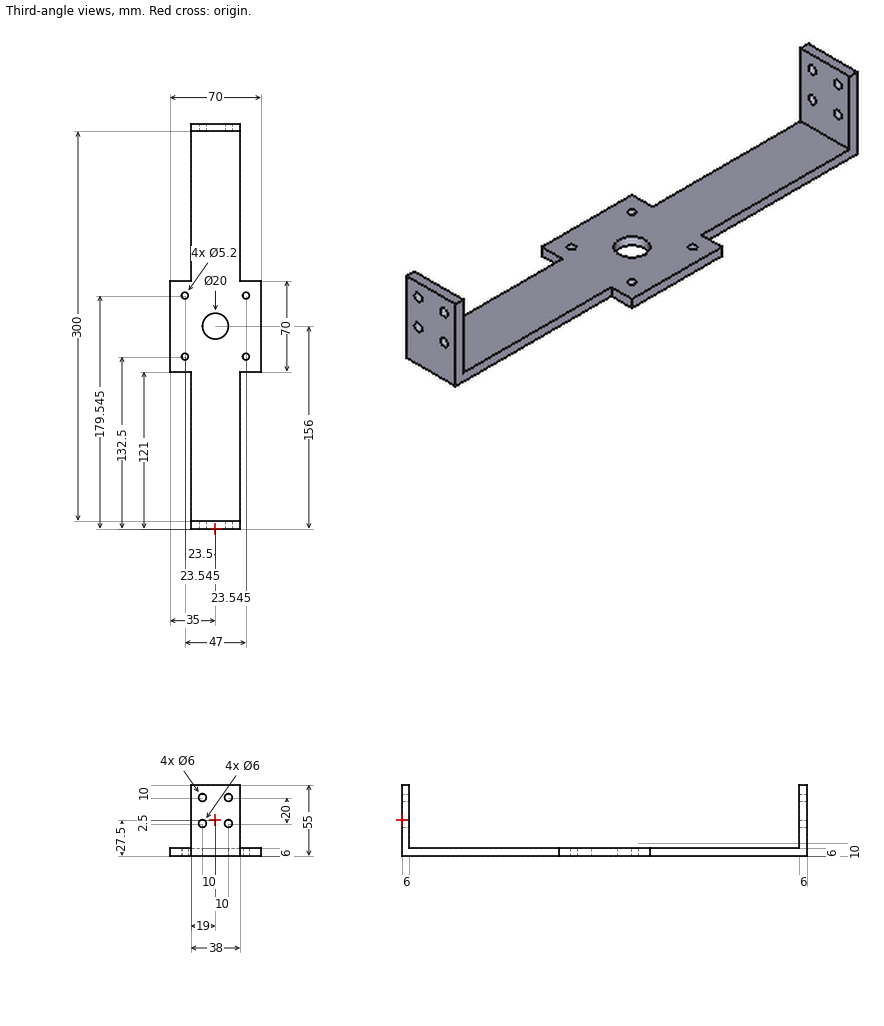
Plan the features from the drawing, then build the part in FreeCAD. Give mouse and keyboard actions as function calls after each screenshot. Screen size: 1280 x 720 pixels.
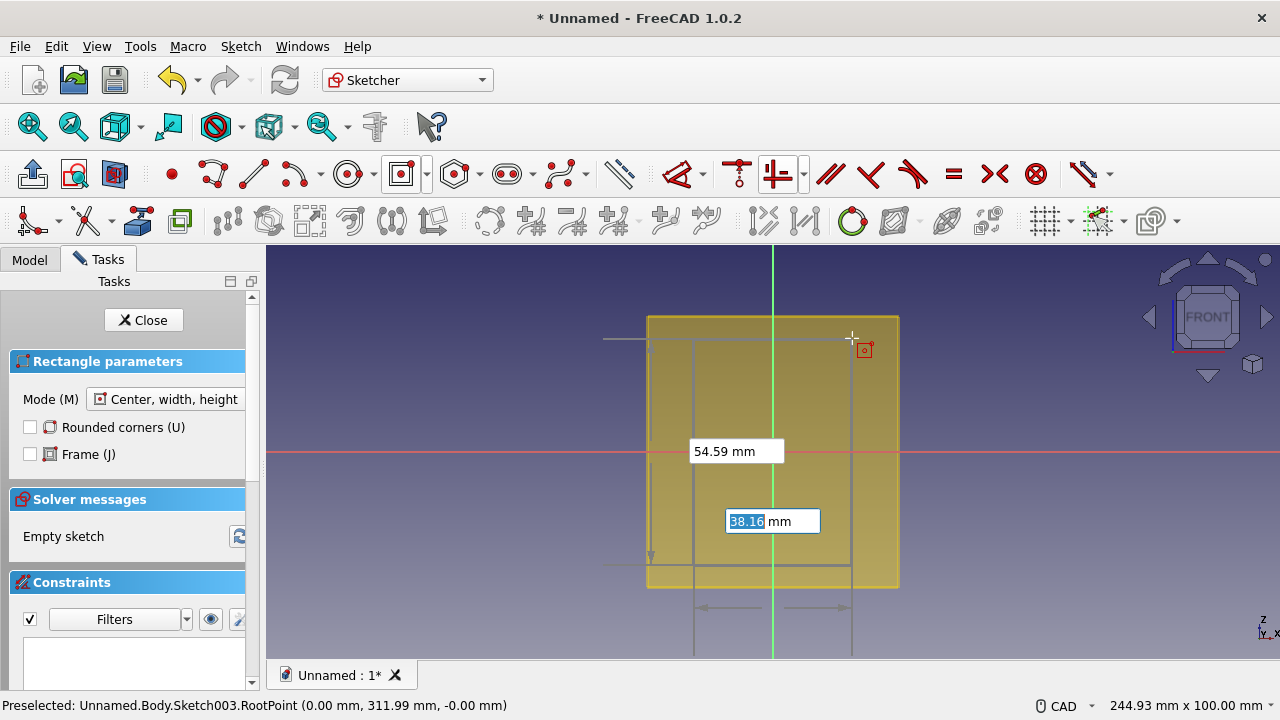
text(38)
key(Tab)
text(55)
key(Return)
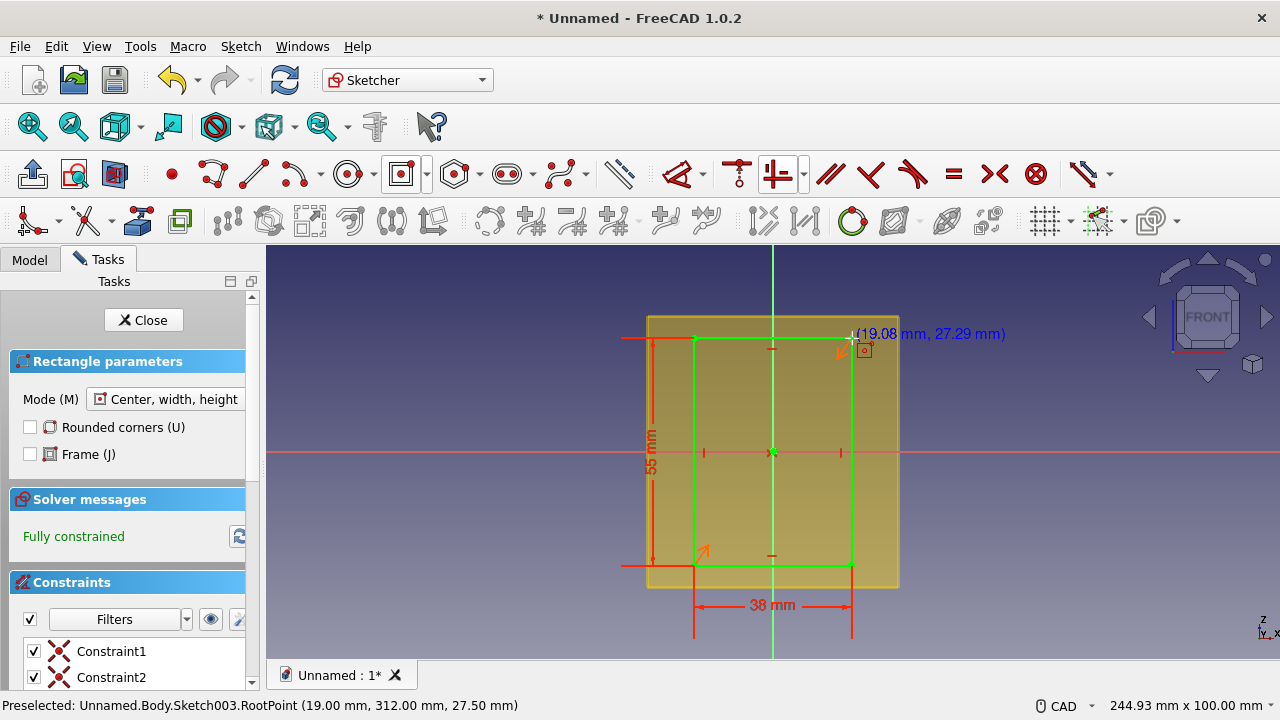
click(348, 174)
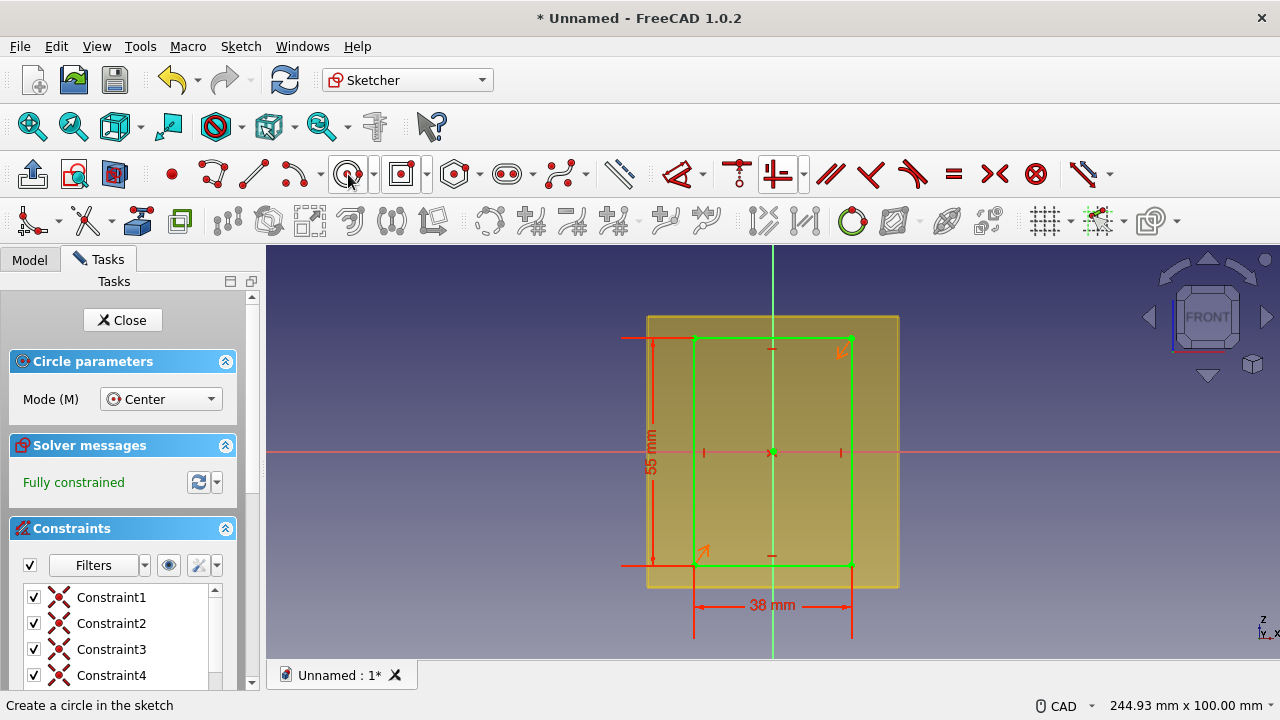
scroll(732, 380, up, 4)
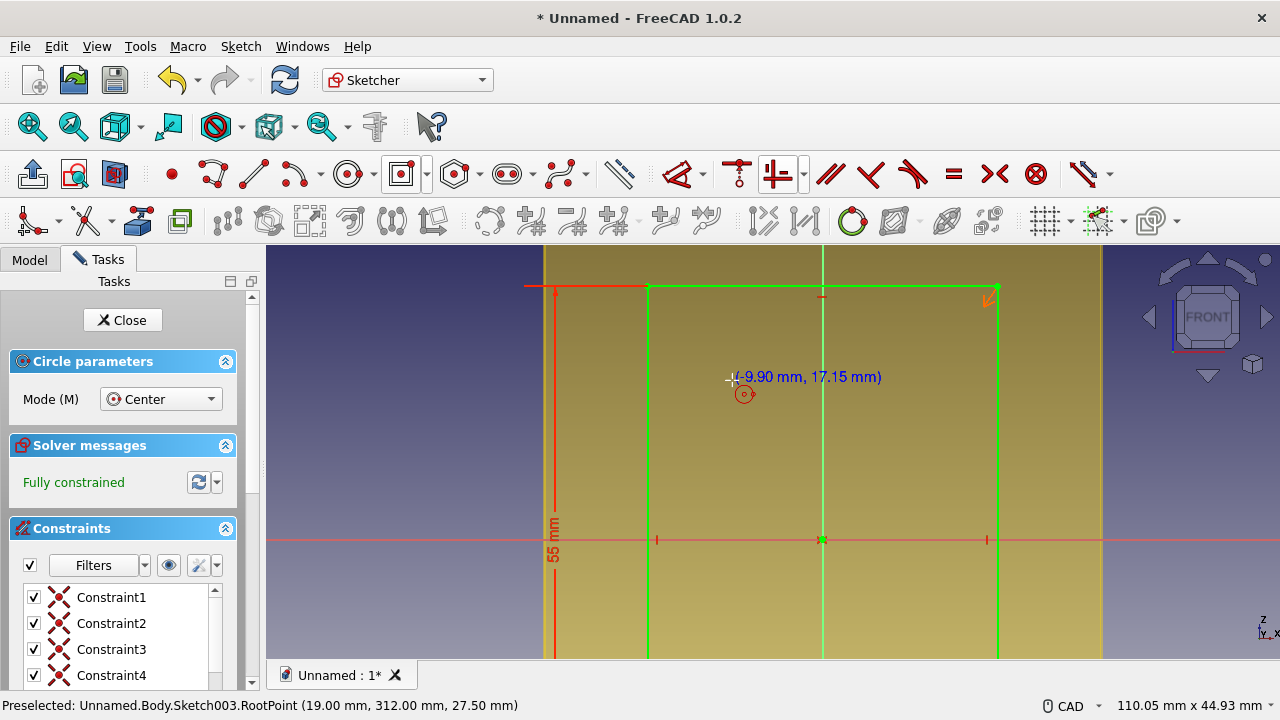
click(731, 379)
move(750, 359)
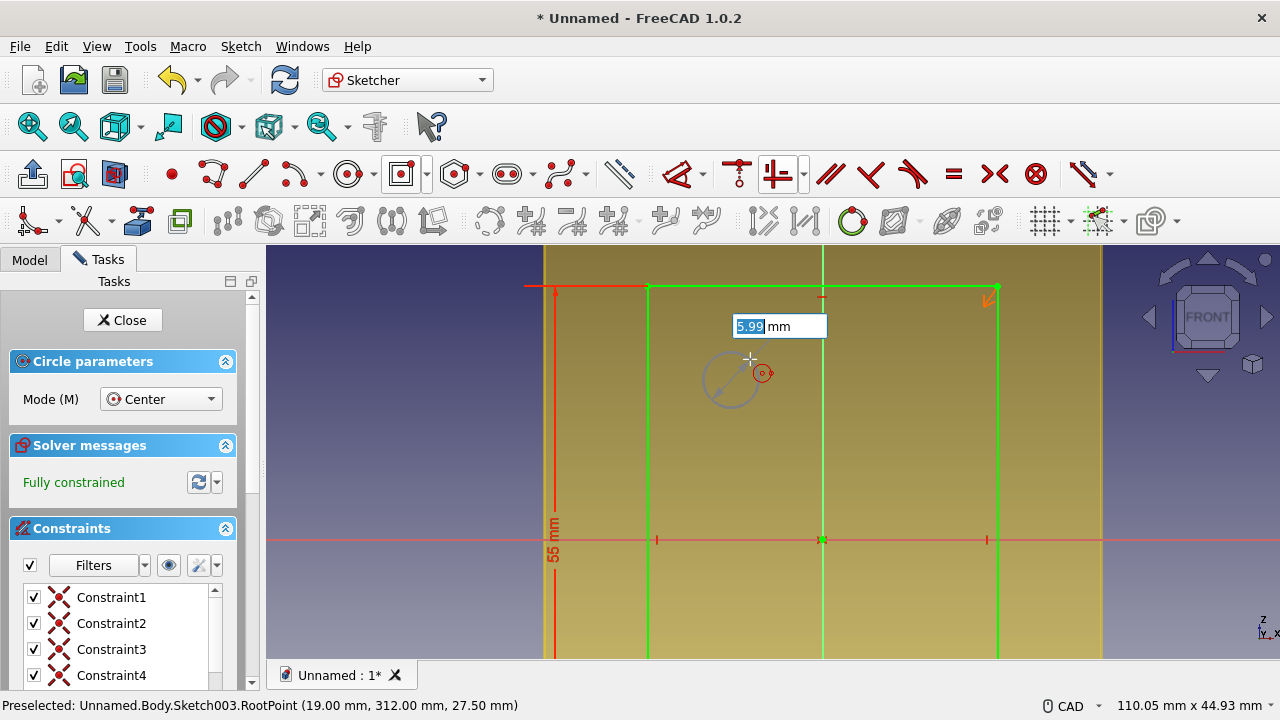
text(6)
key(Return)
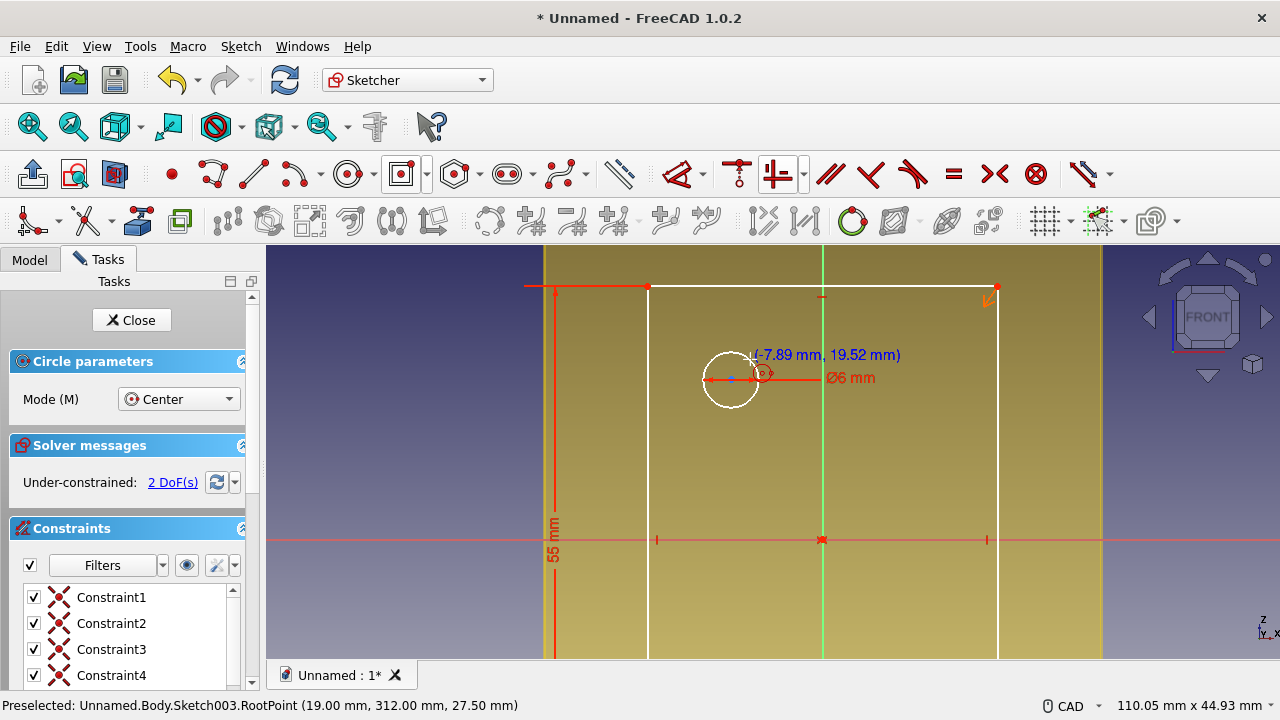
click(915, 379)
move(934, 359)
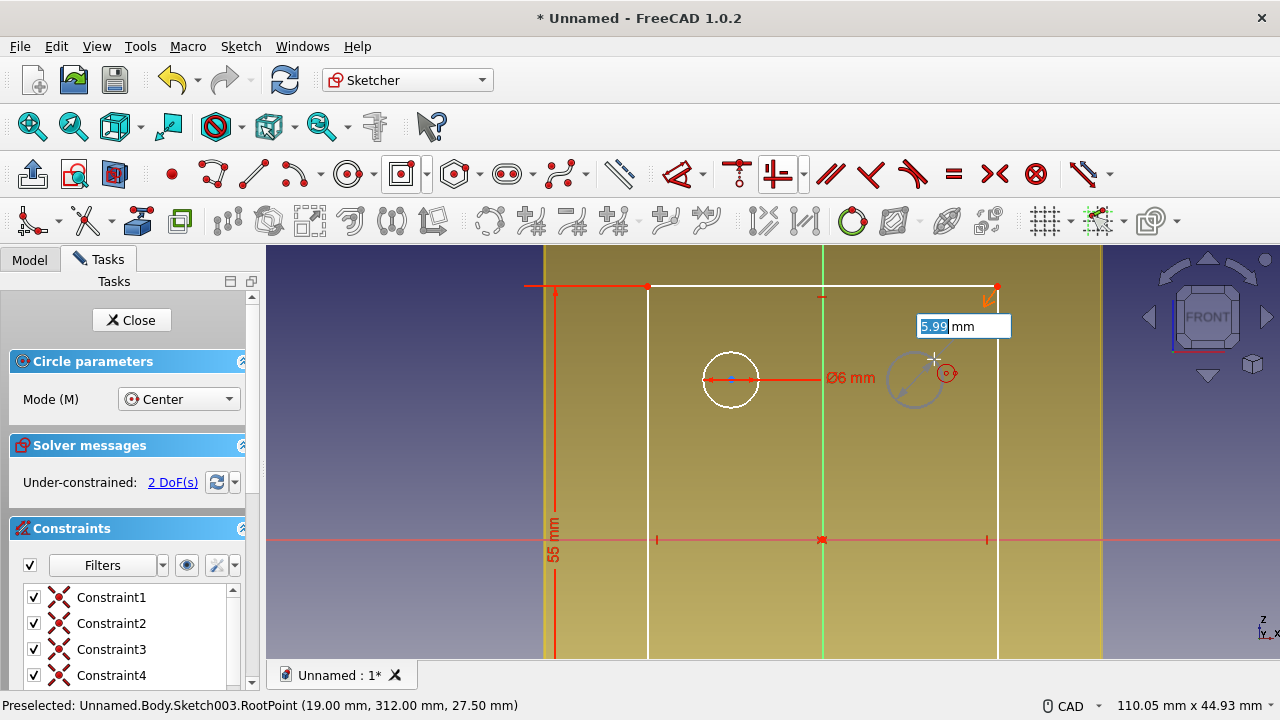
text(6)
key(Return)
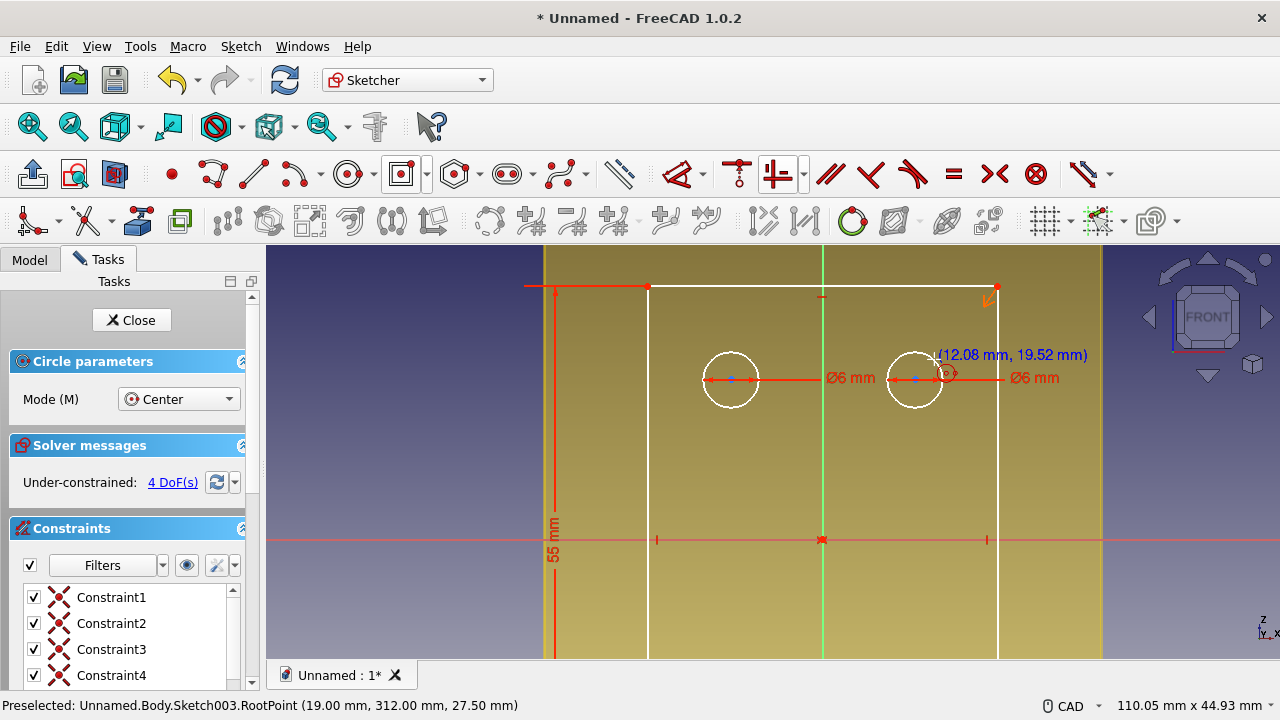
click(731, 563)
move(750, 582)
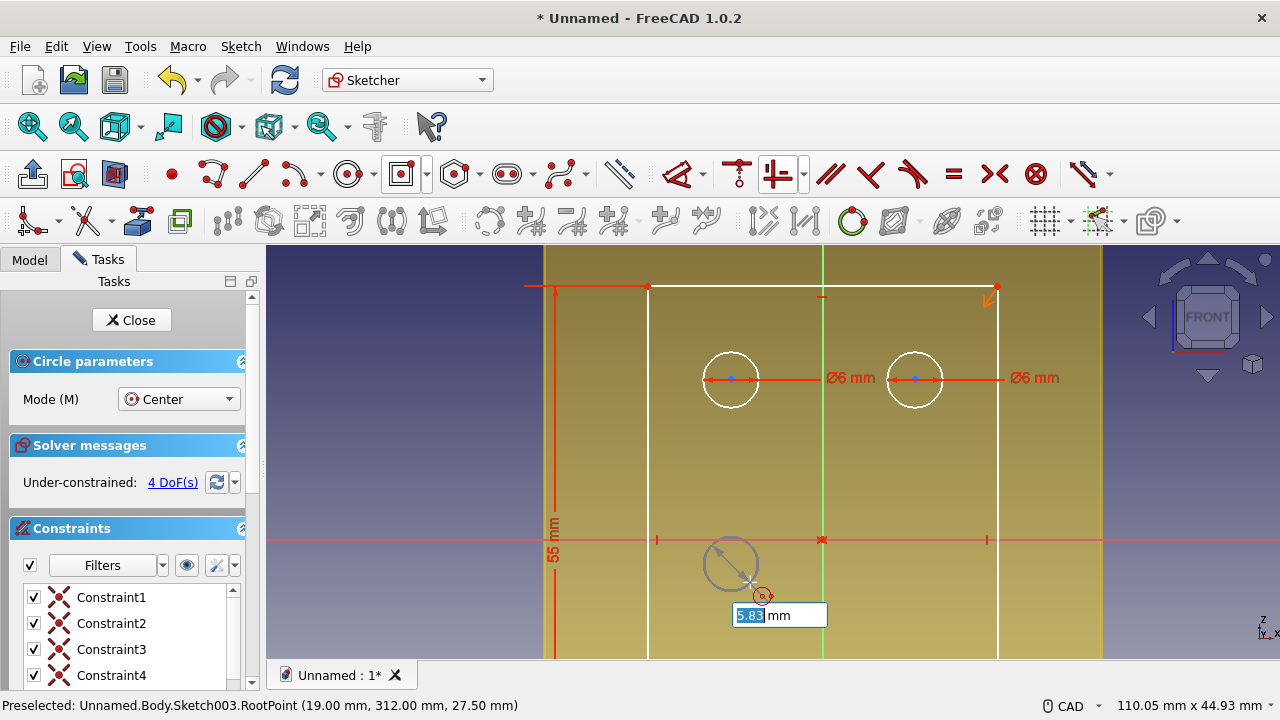
text(6)
key(Return)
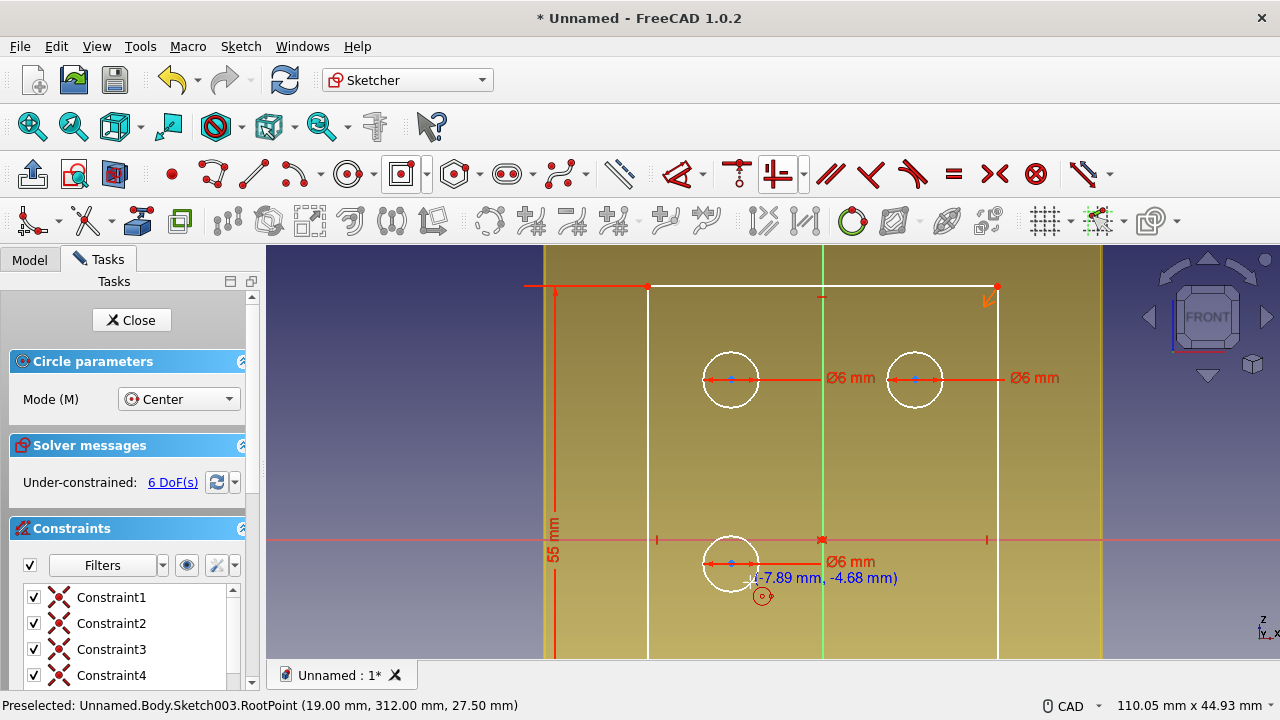
click(915, 563)
move(934, 582)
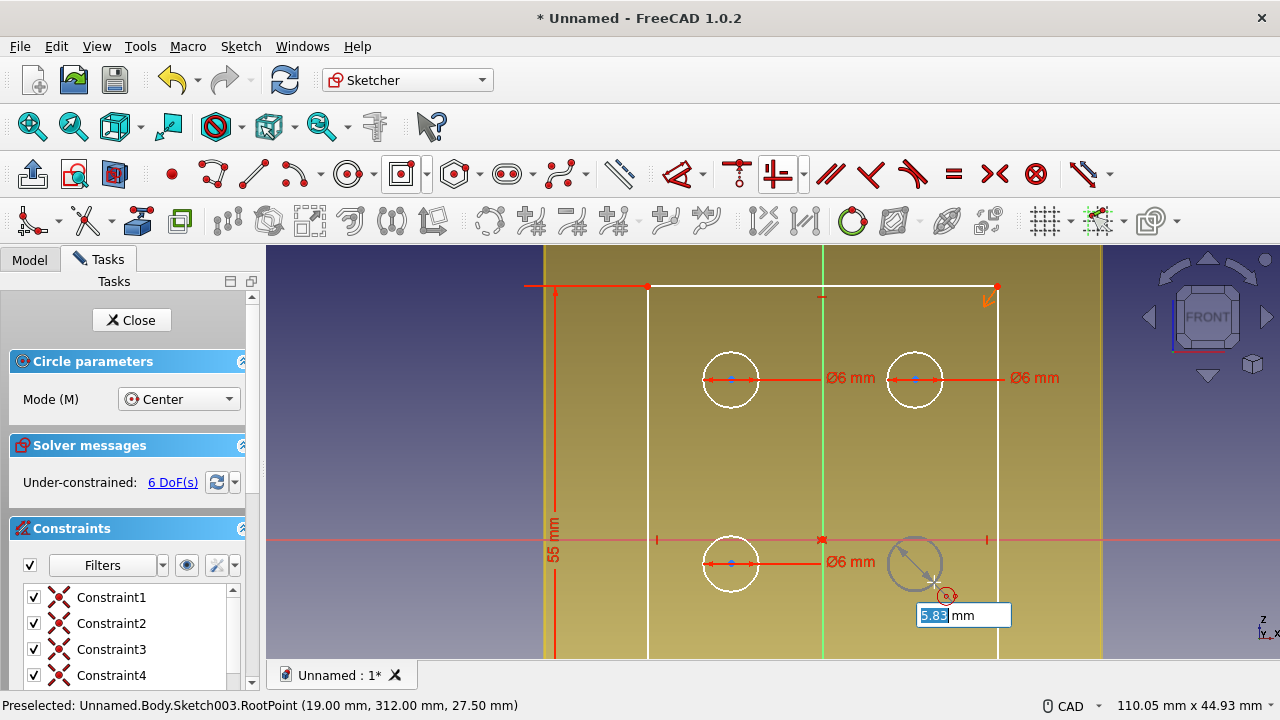
text(6)
key(Return)
key(Escape)